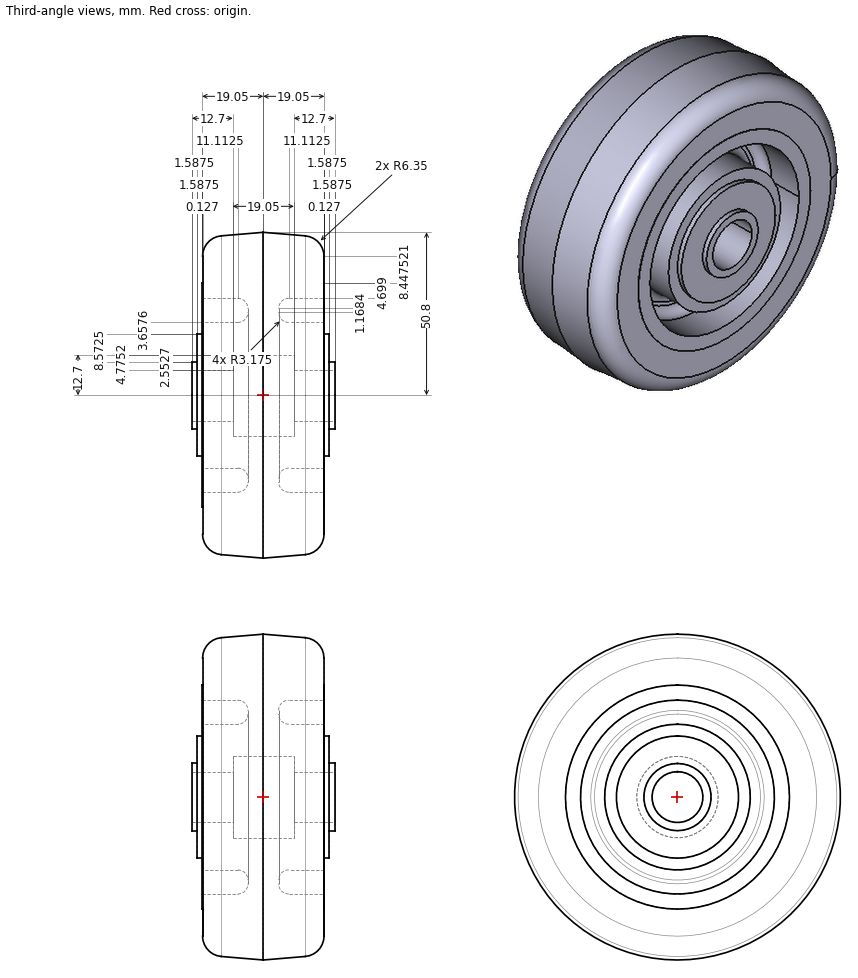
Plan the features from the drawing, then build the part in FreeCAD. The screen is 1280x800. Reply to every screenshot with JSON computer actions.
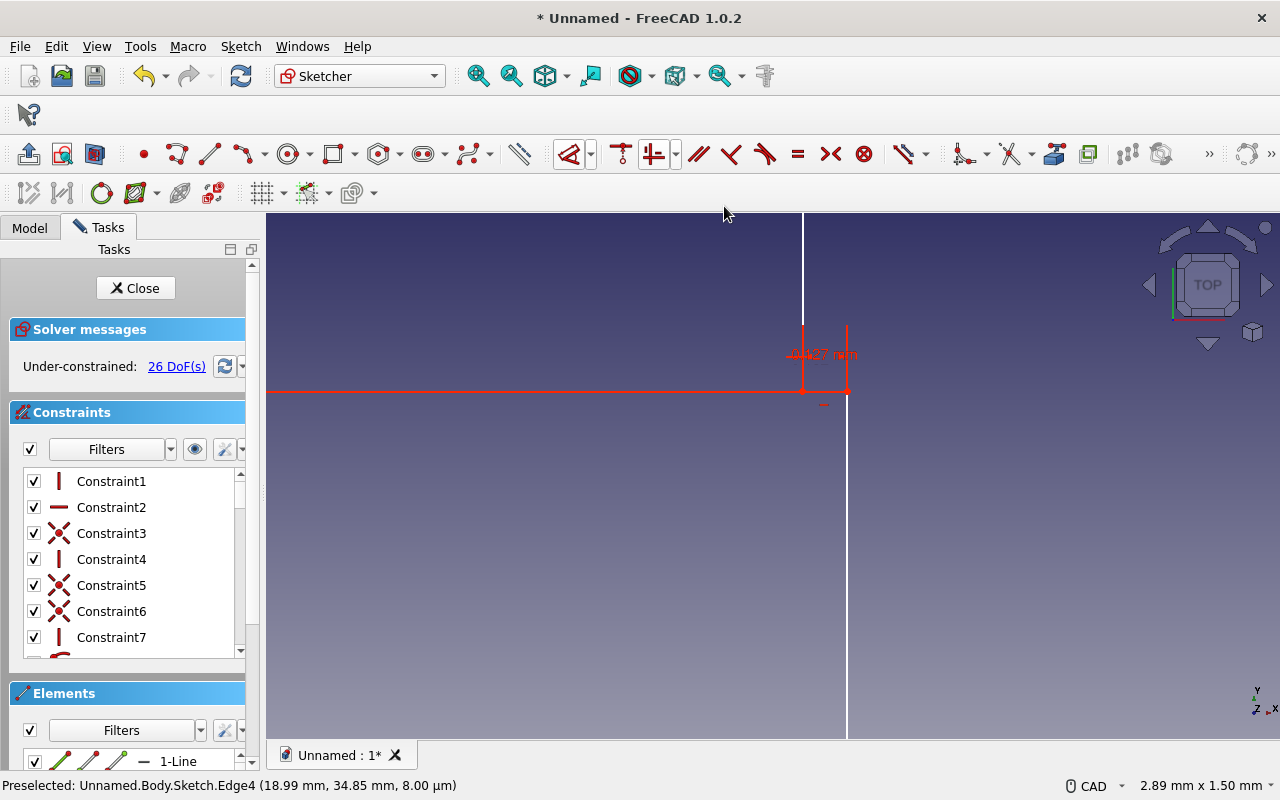
{"action": "scroll", "coordinate": [704, 476], "scroll_direction": "down", "scroll_amount": 15}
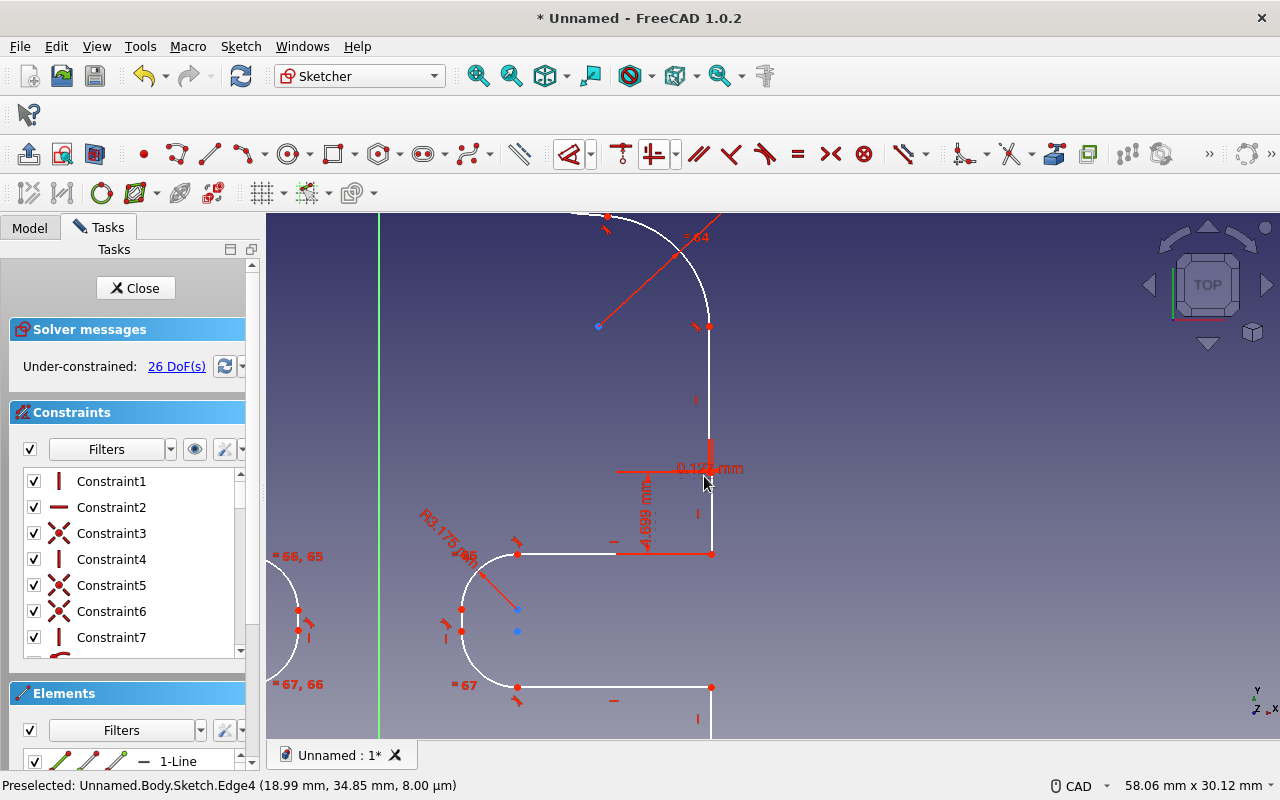
{"action": "scroll", "coordinate": [894, 382], "scroll_direction": "down", "scroll_amount": 5}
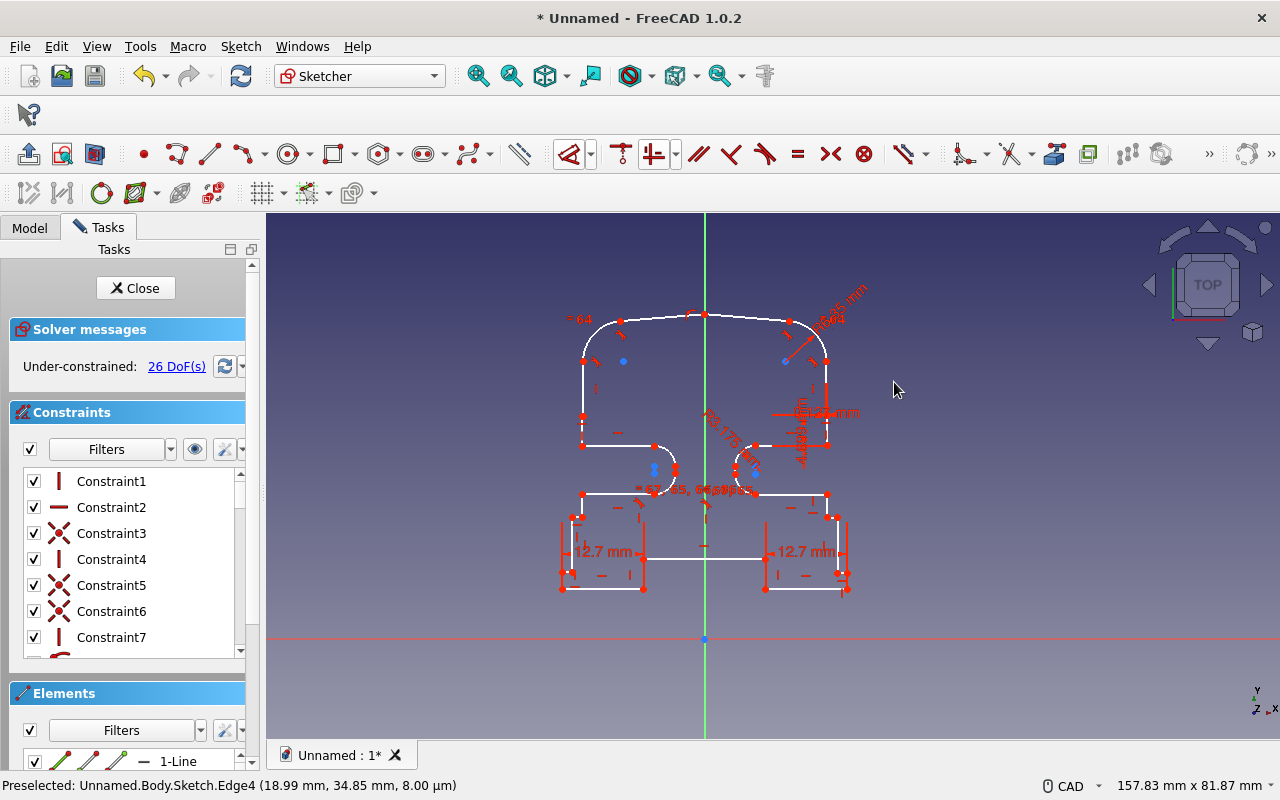
{"action": "scroll", "coordinate": [583, 416], "scroll_direction": "up", "scroll_amount": 20}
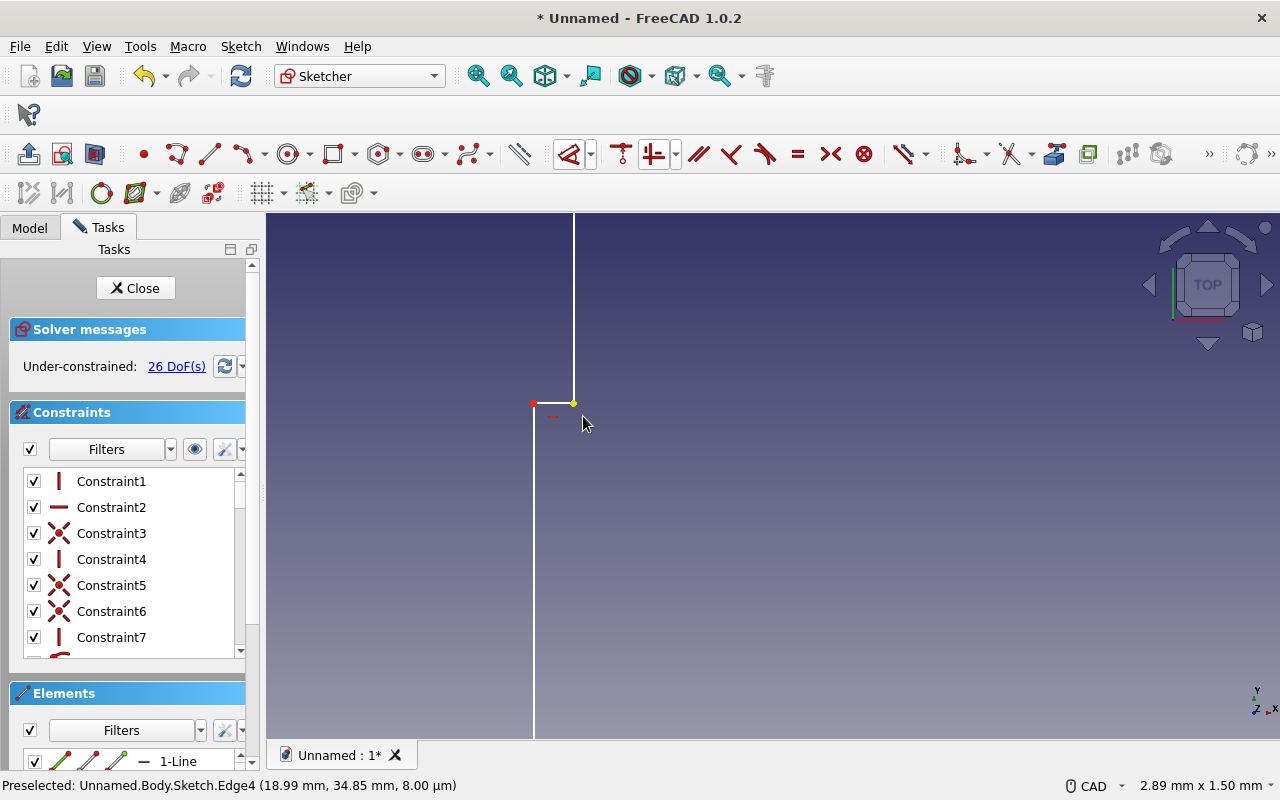
{"action": "left_click", "coordinate": [562, 403]}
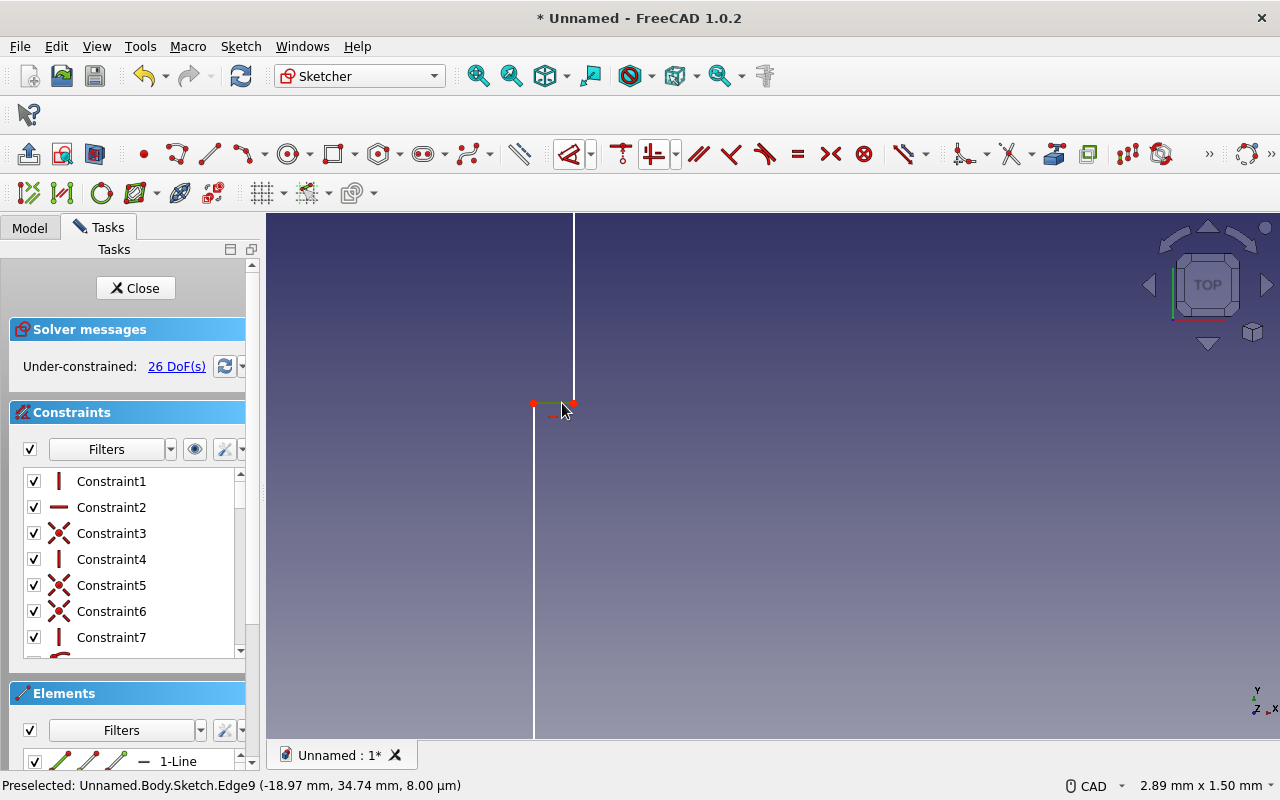
{"action": "left_click", "coordinate": [590, 154]}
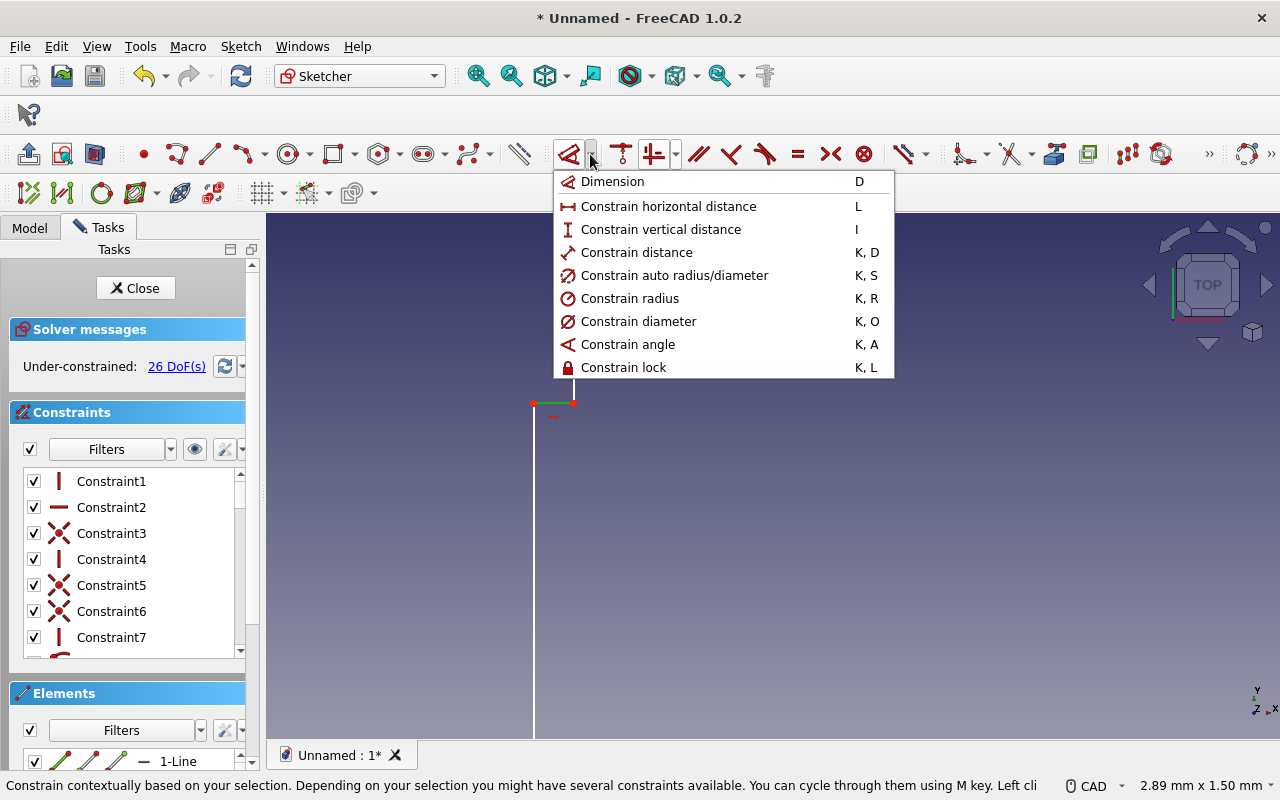
{"action": "left_click", "coordinate": [724, 206]}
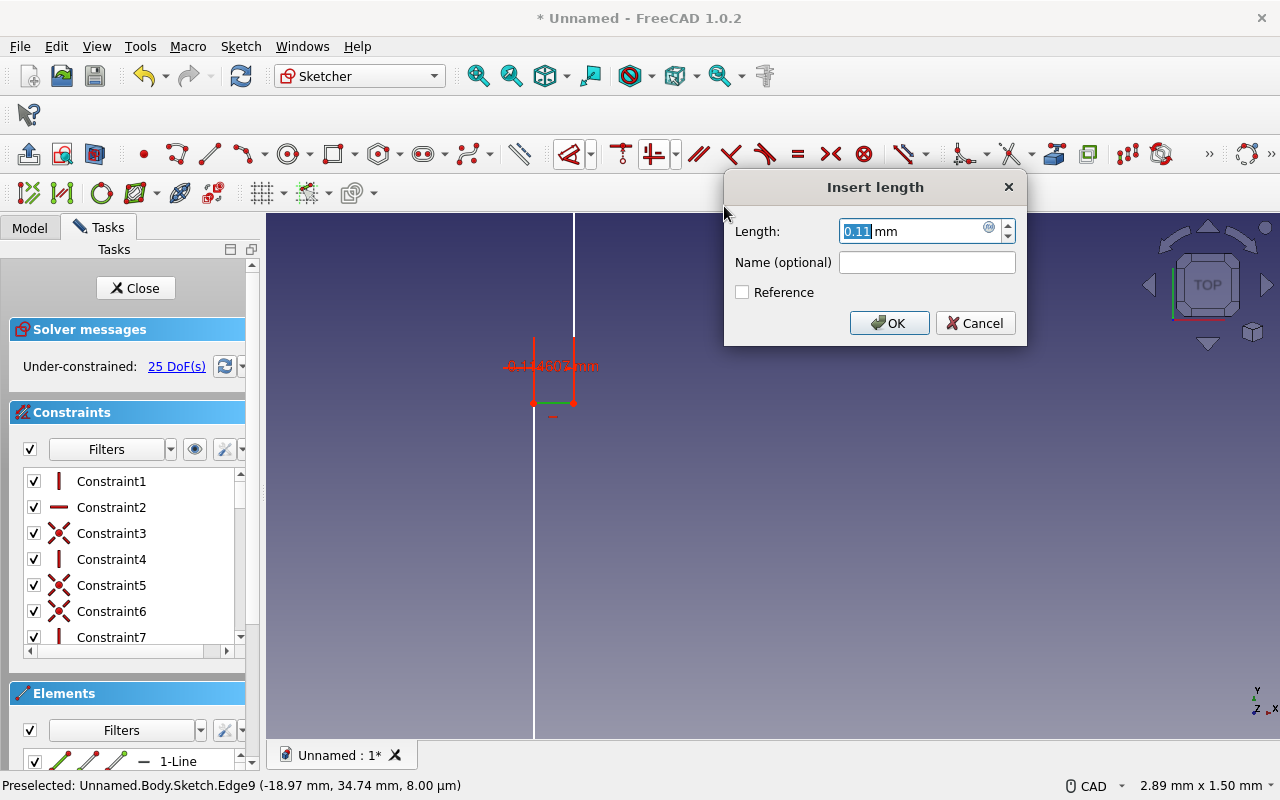
{"action": "type", "text": "0.127"}
{"action": "key", "text": "Return"}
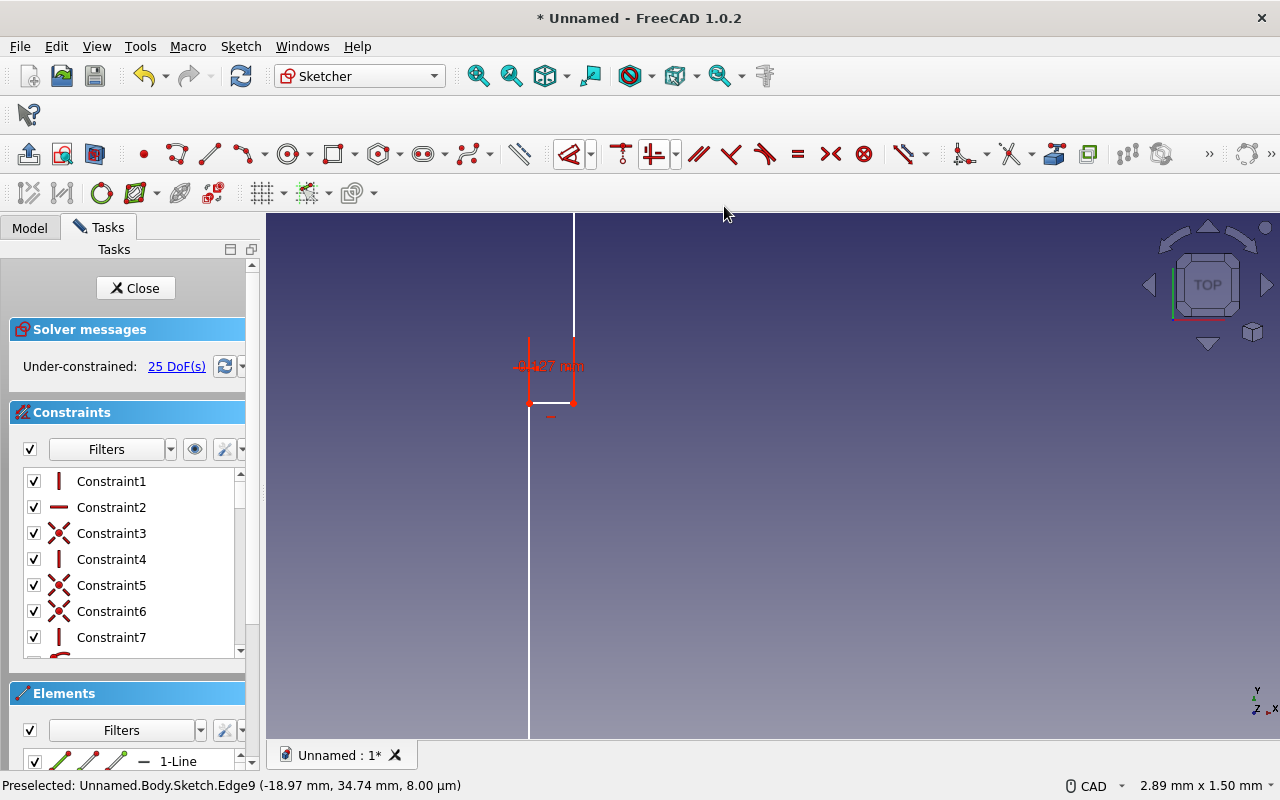
{"action": "scroll", "coordinate": [704, 476], "scroll_direction": "down", "scroll_amount": 15}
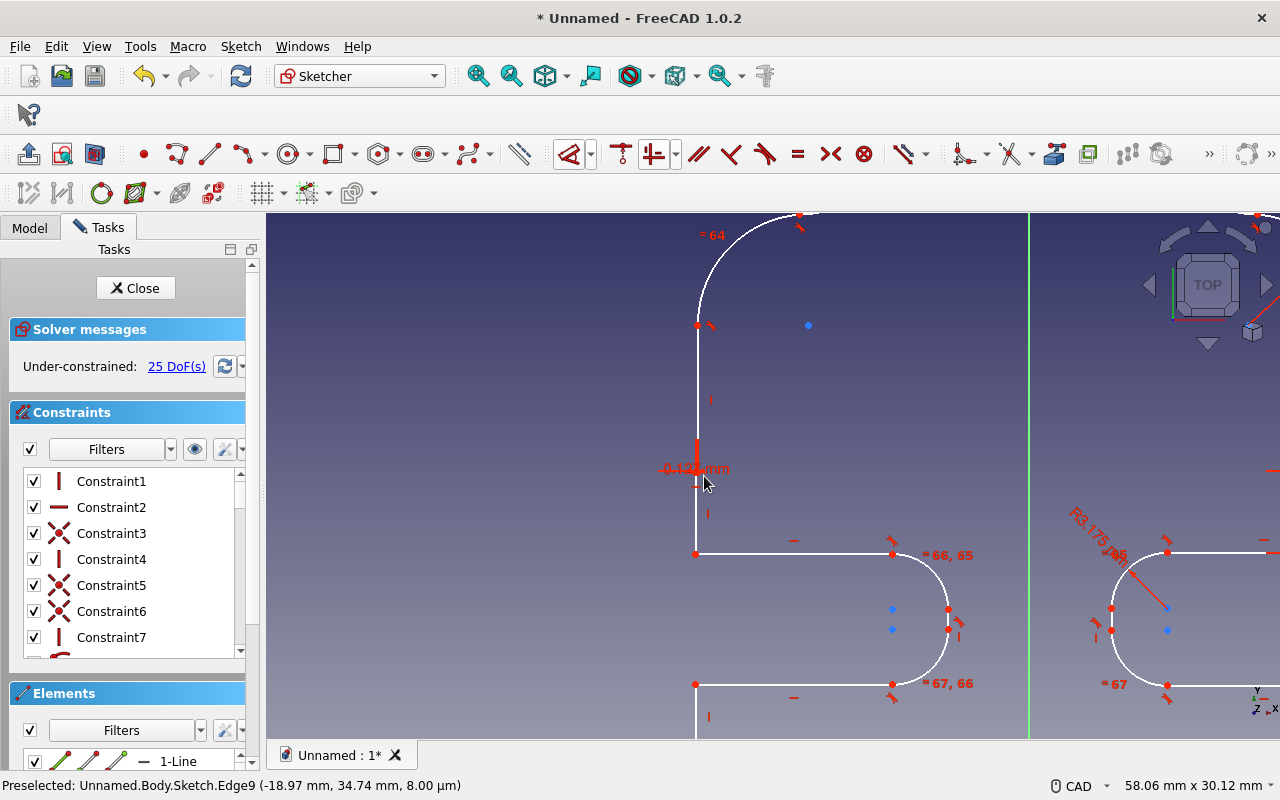
{"action": "scroll", "coordinate": [516, 383], "scroll_direction": "down", "scroll_amount": 5}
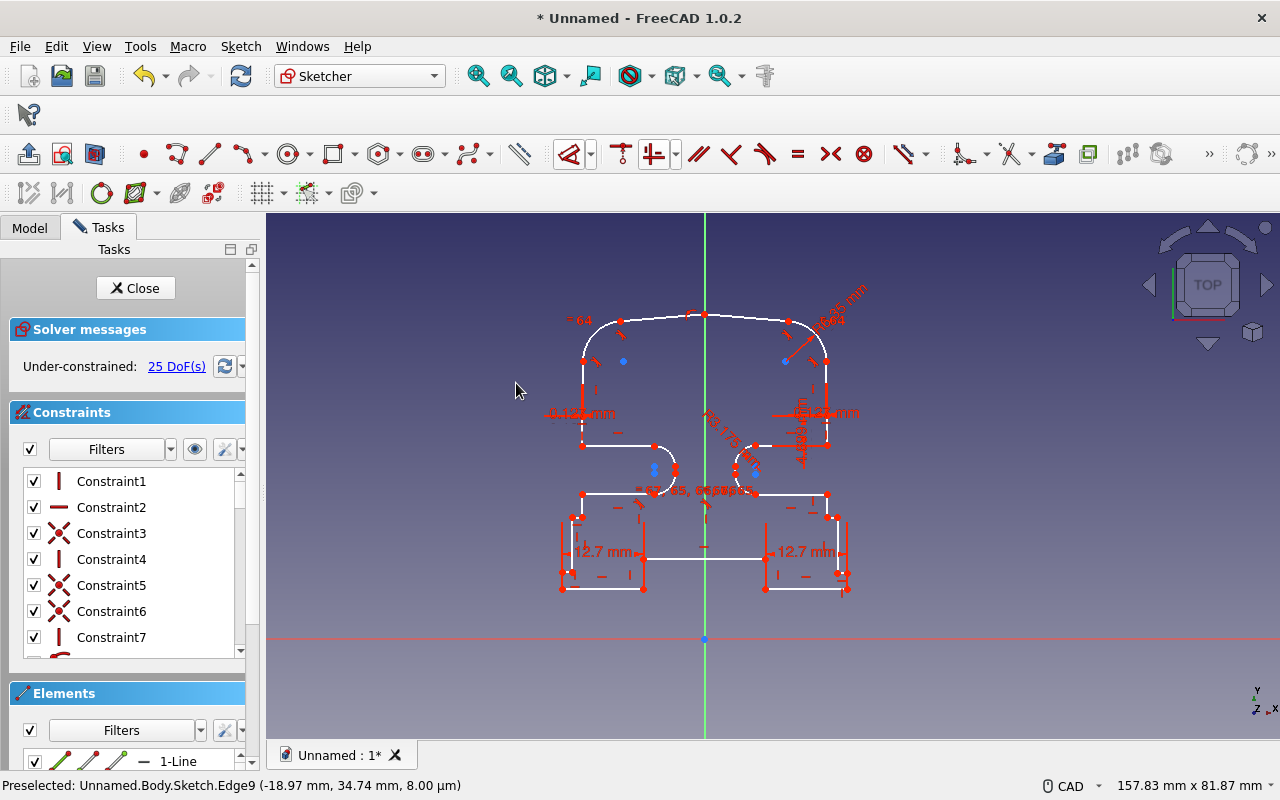
{"action": "scroll", "coordinate": [582, 425], "scroll_direction": "up", "scroll_amount": 3}